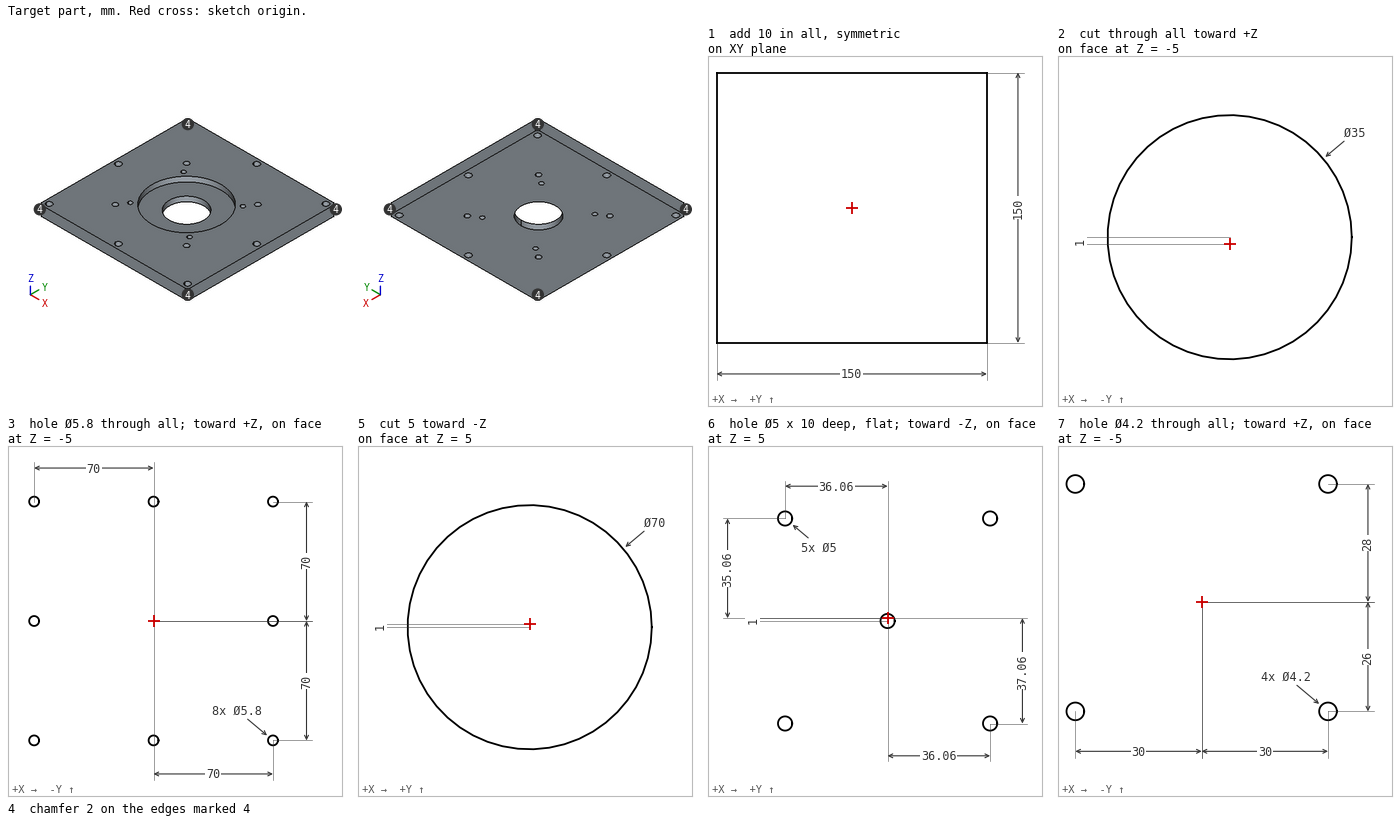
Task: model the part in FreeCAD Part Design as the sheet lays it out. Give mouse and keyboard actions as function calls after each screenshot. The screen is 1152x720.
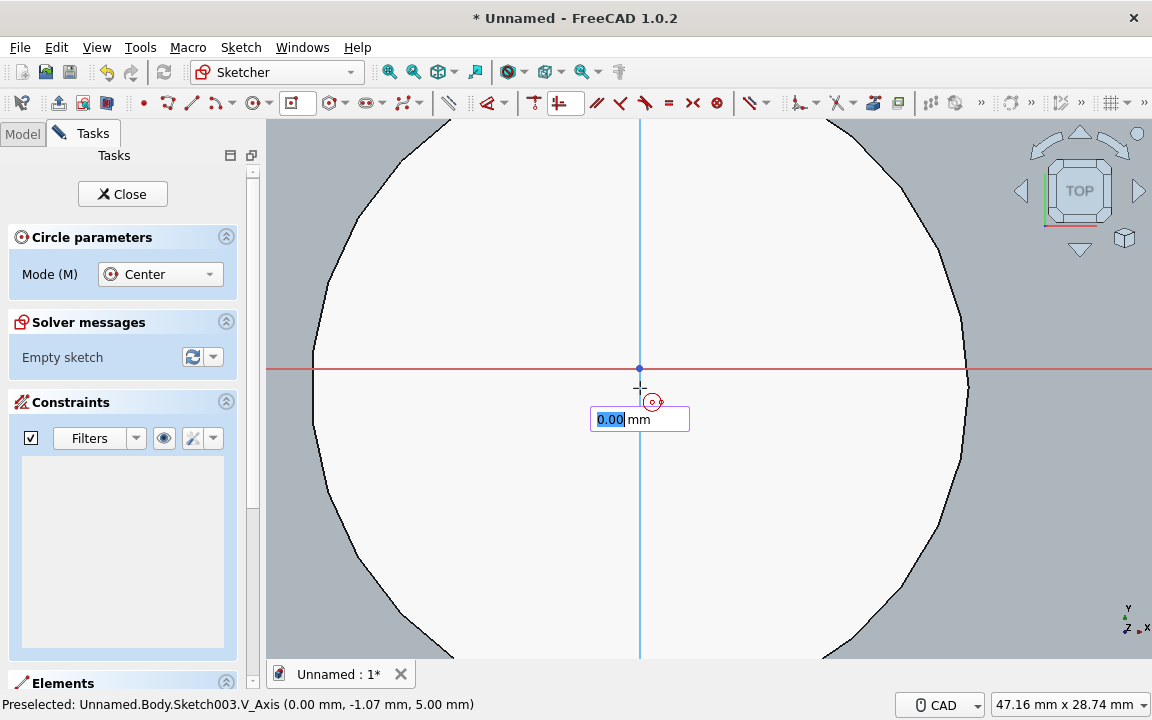
scroll(641, 389, down, 7)
move(756, 274)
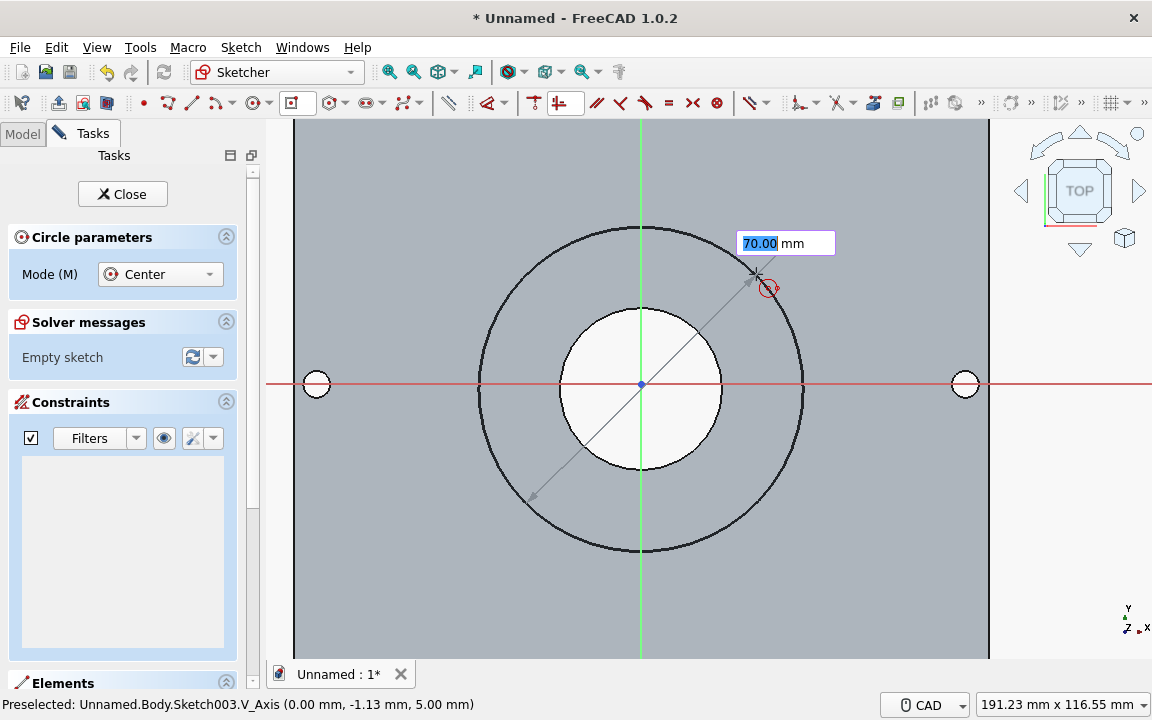
text(70)
key(Return)
key(Escape)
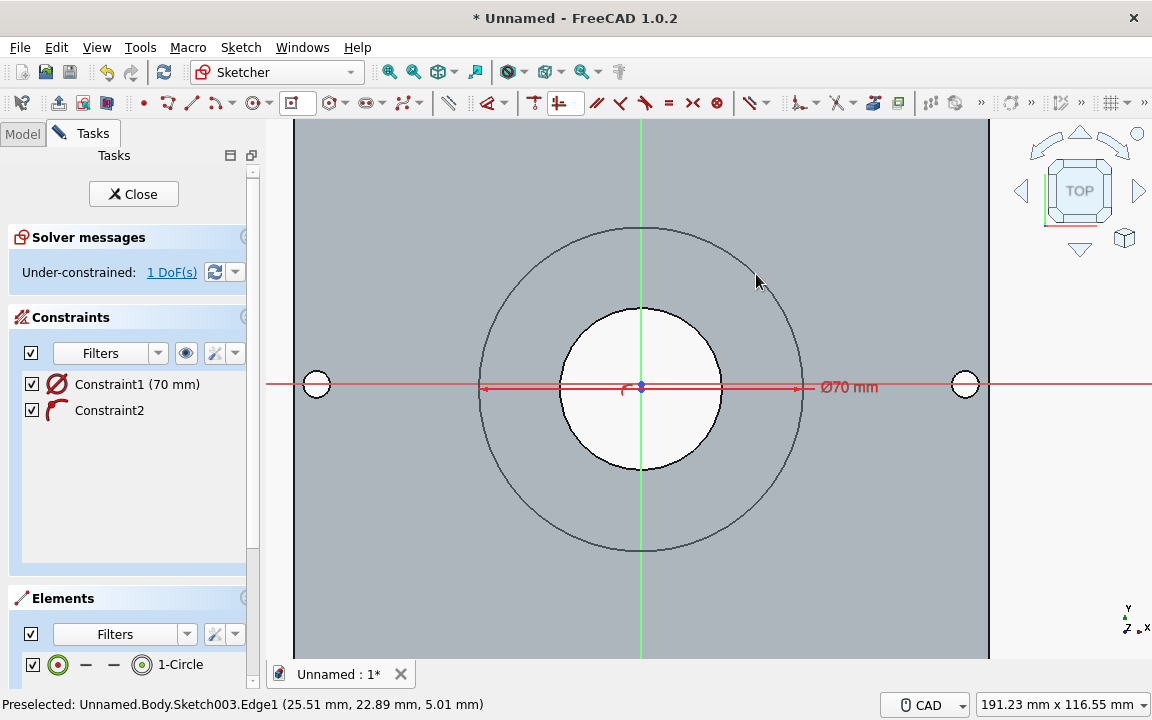
key(d)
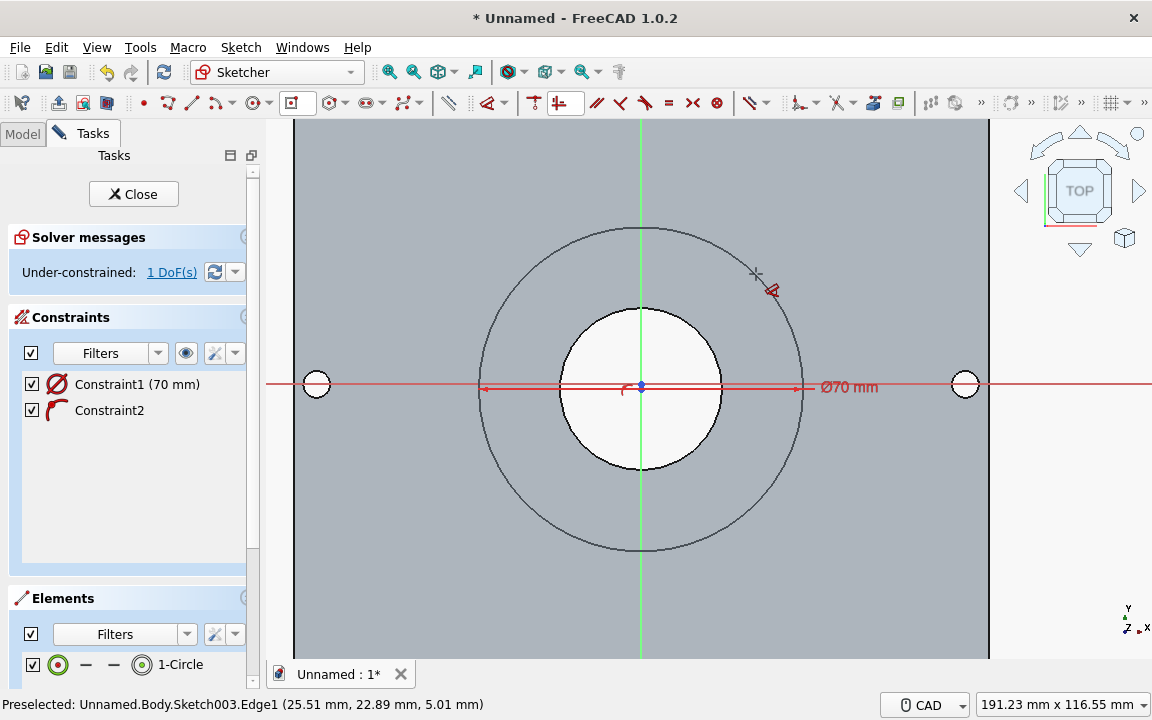
scroll(641, 389, up, 11)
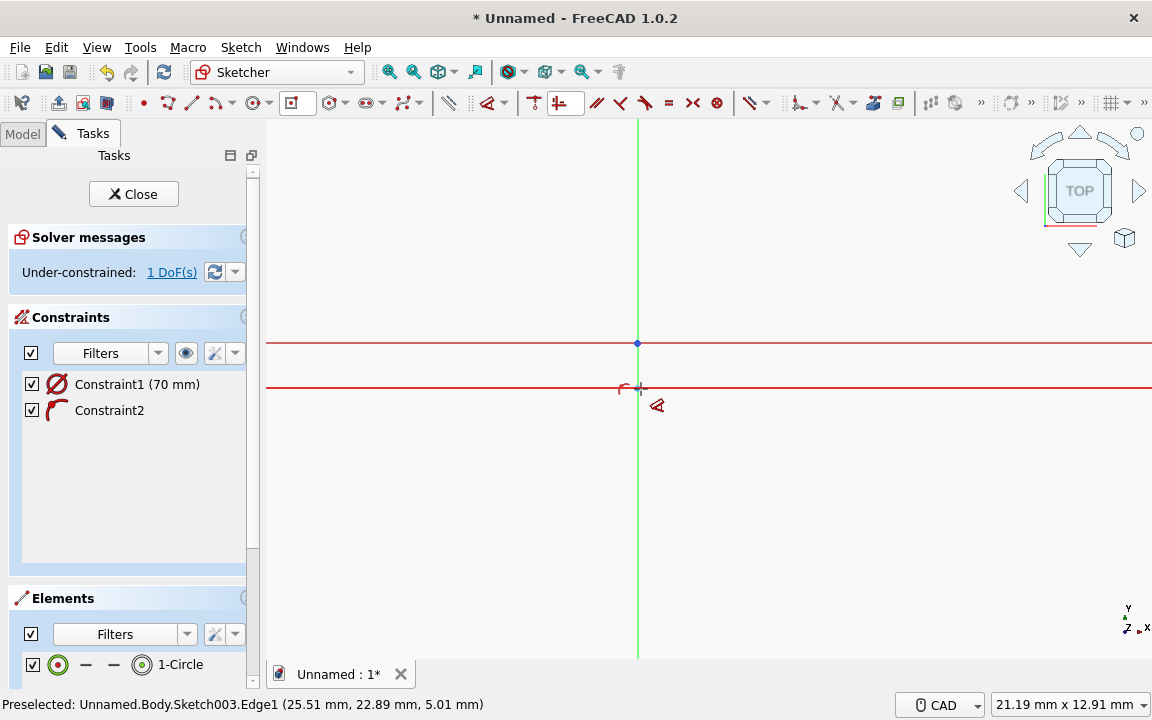
click(638, 388)
click(672, 366)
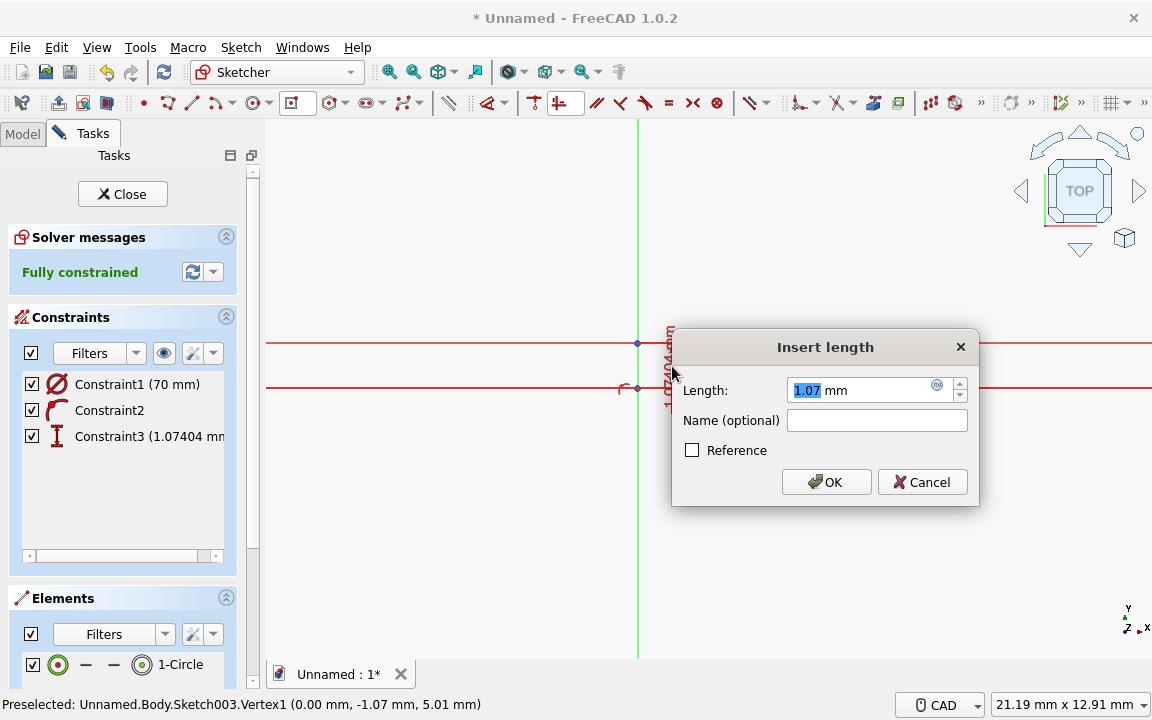
text(1)
key(Return)
key(Escape)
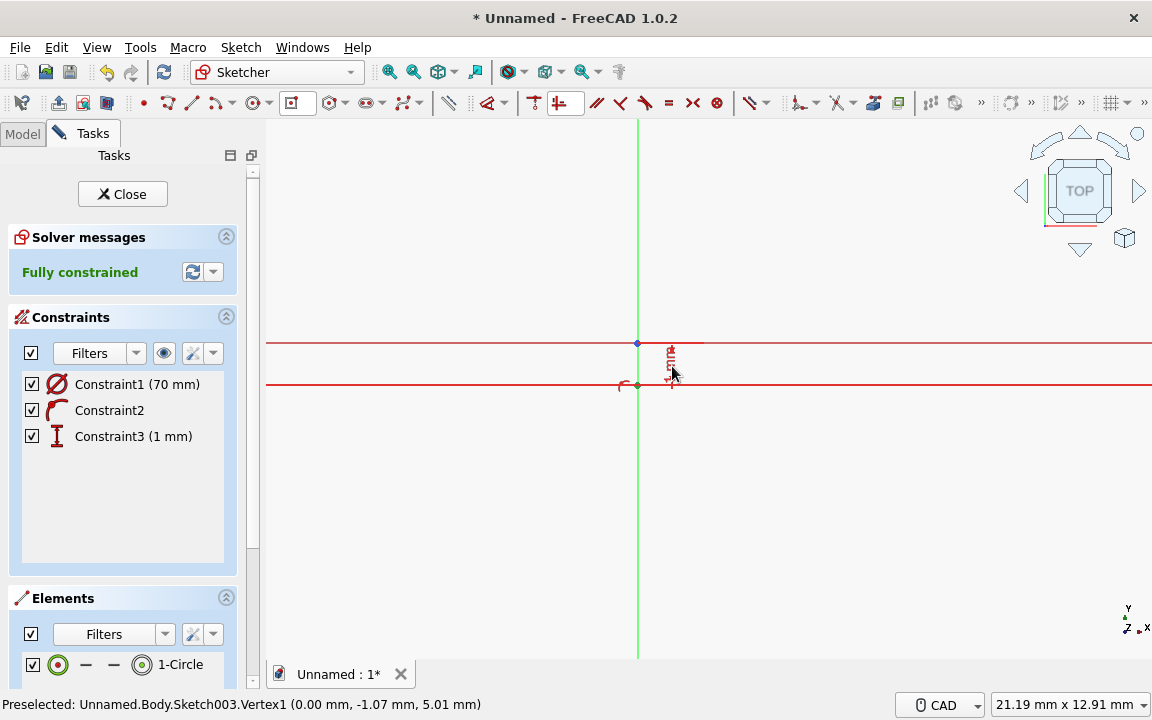
click(123, 194)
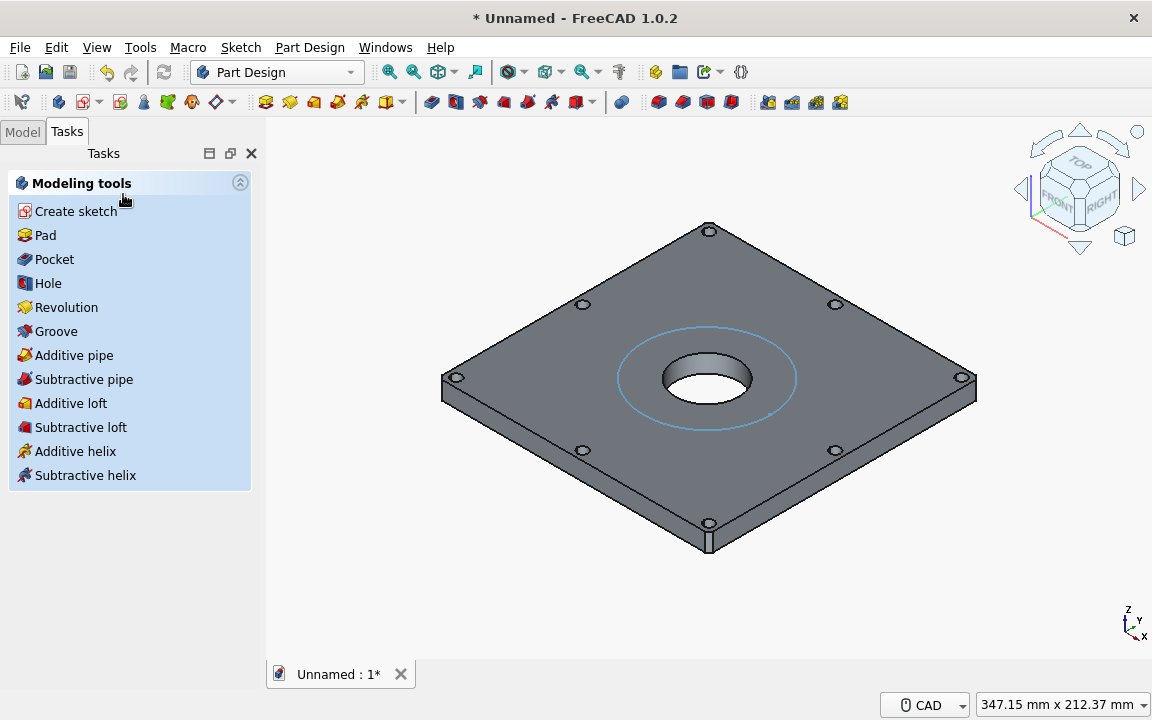
click(432, 102)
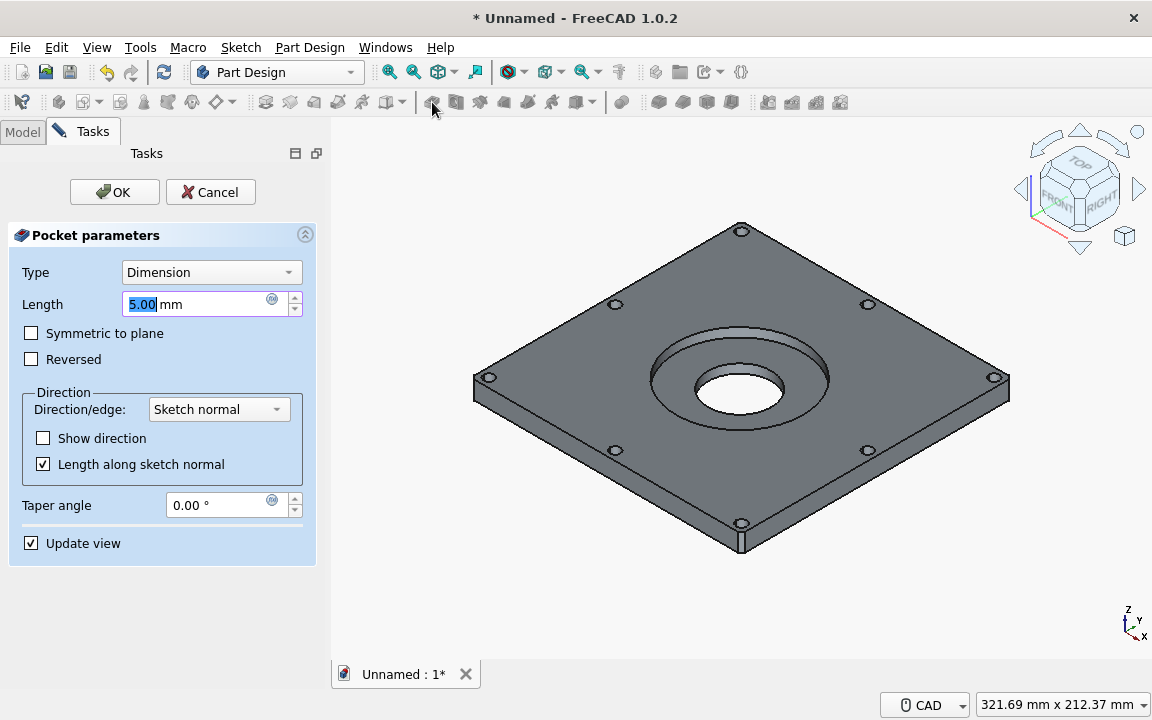
text(5)
key(Tab)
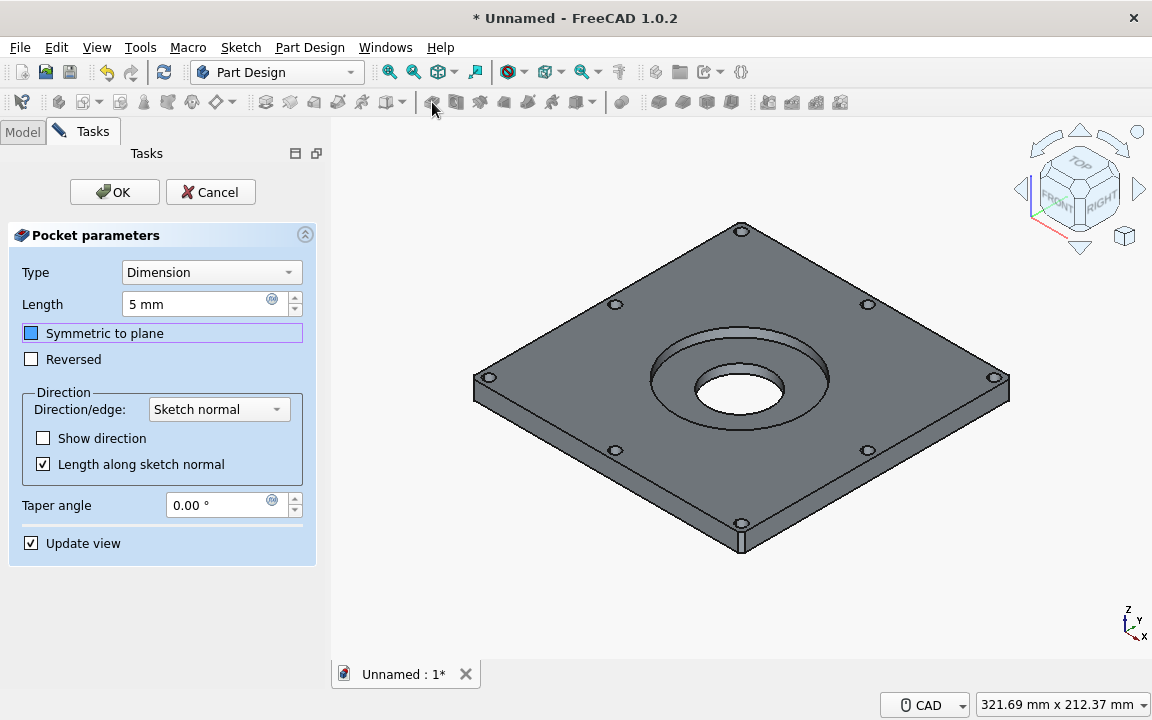
click(115, 192)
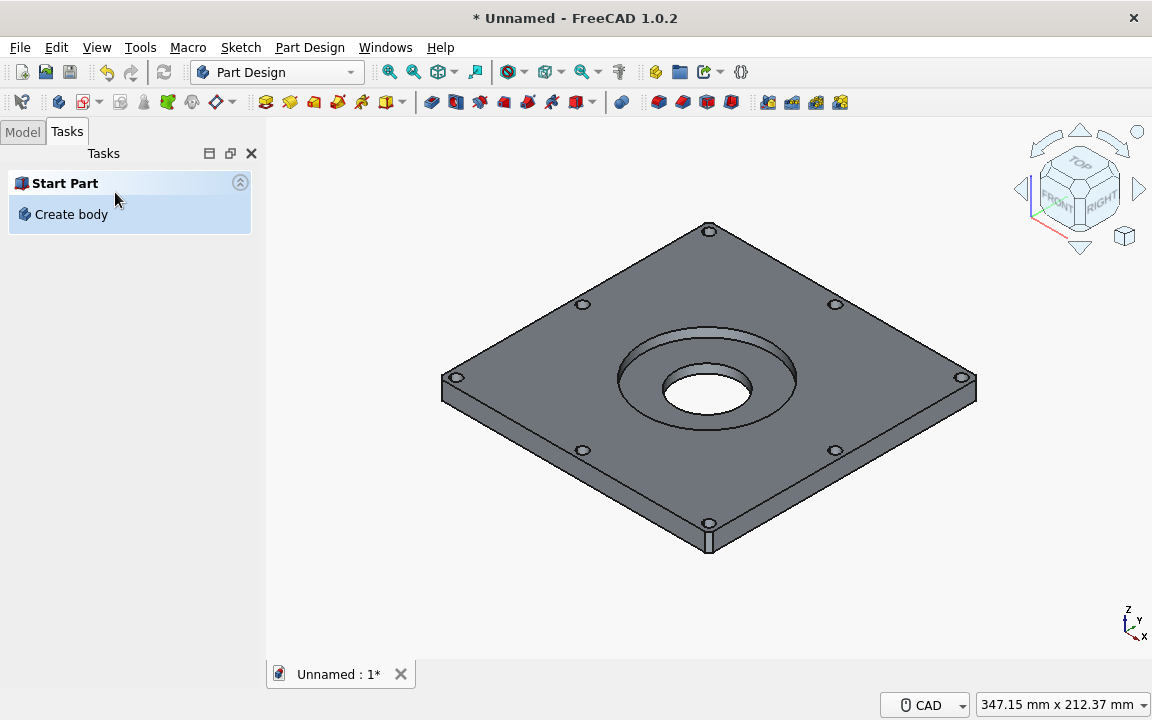
click(864, 377)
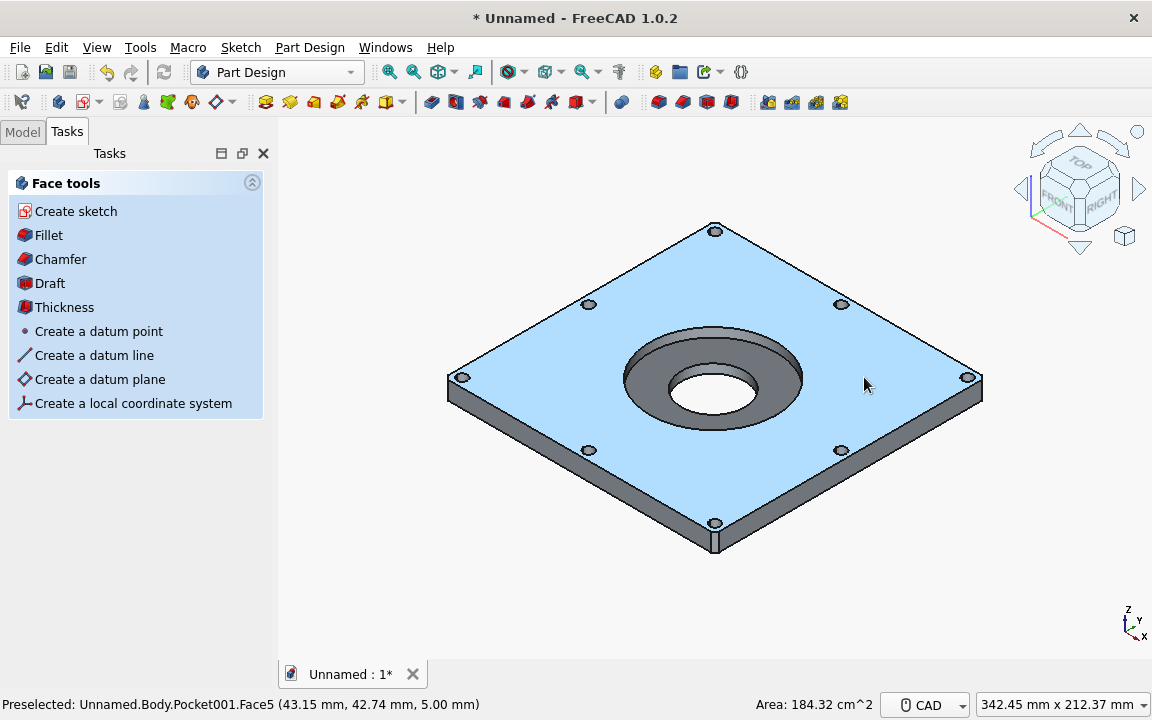
click(84, 102)